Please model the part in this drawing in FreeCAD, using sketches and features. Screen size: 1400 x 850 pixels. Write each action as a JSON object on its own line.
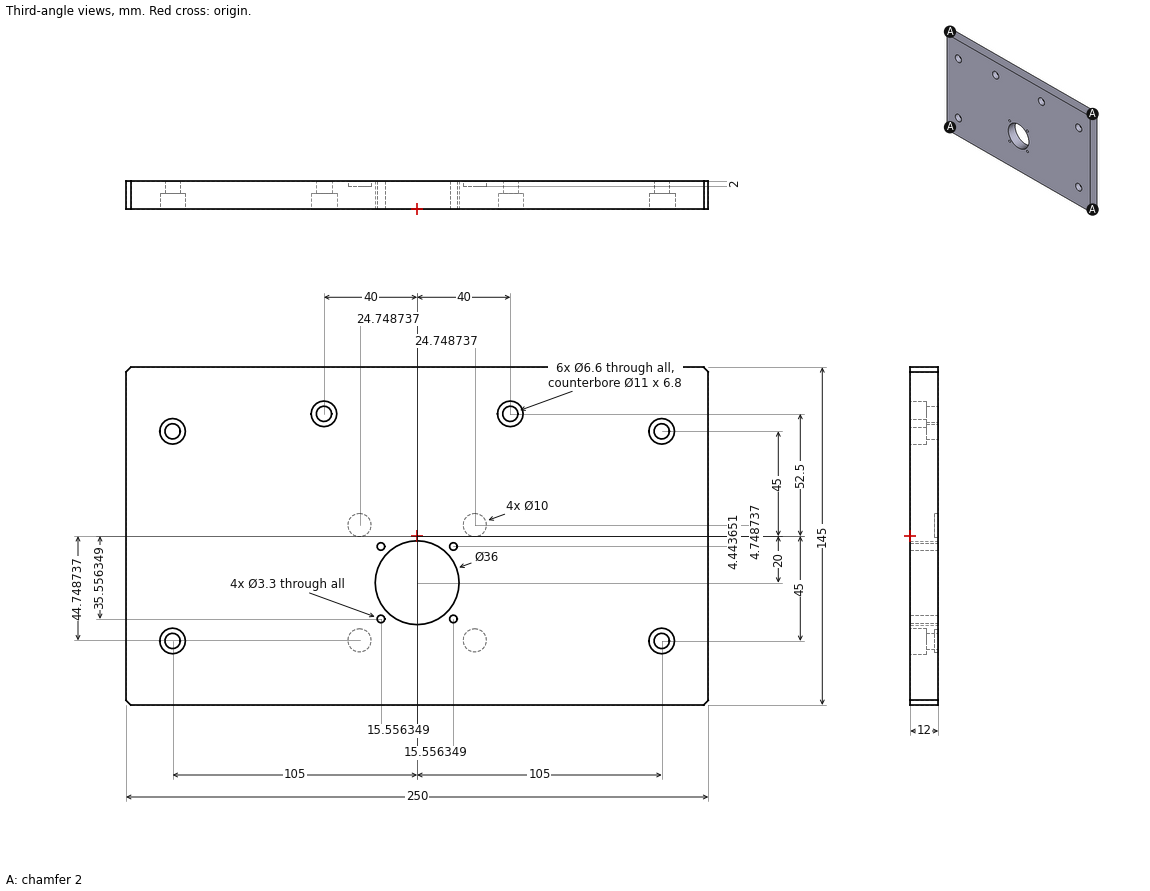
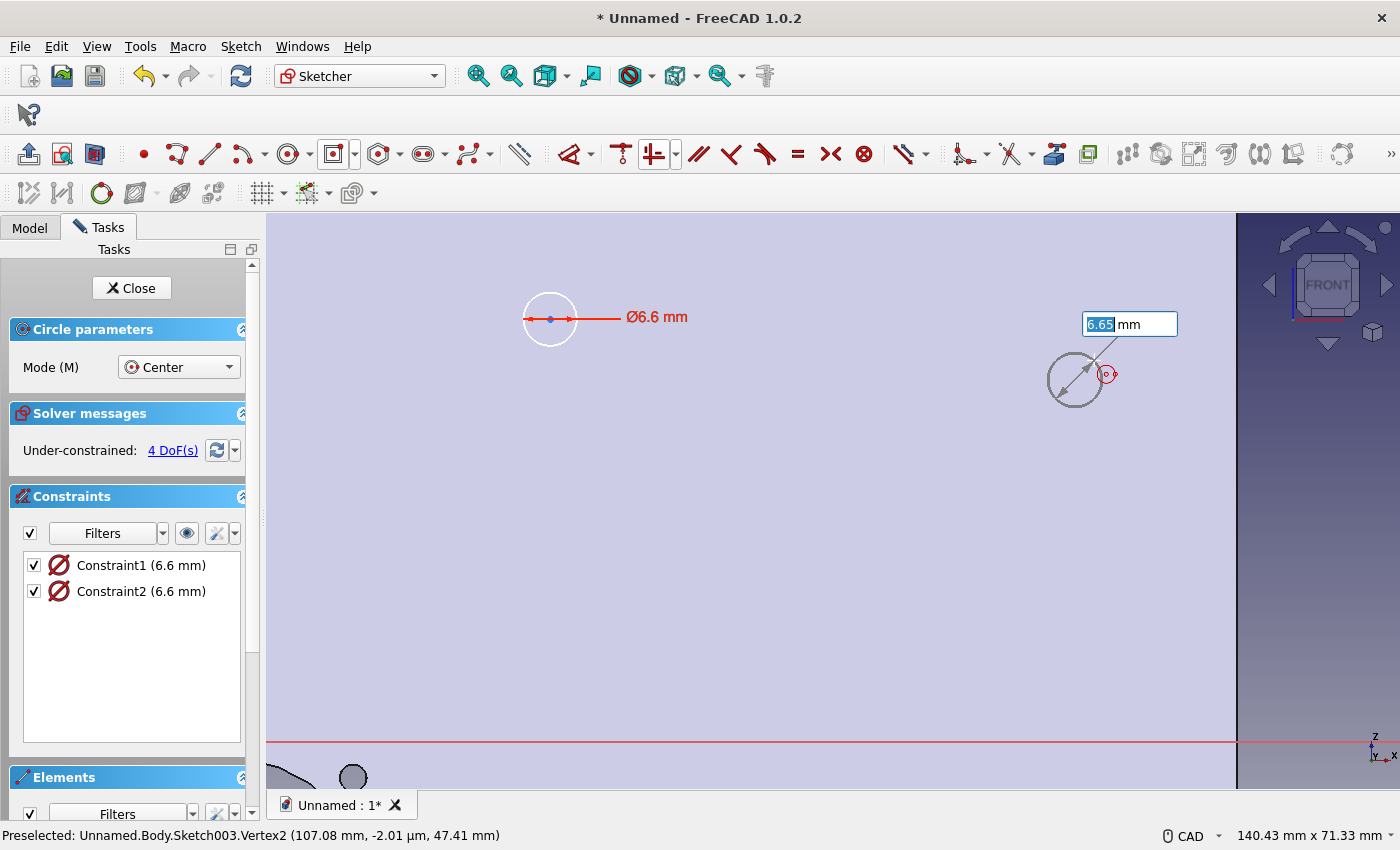
{"action": "type", "text": "6.6"}
{"action": "key", "text": "Return"}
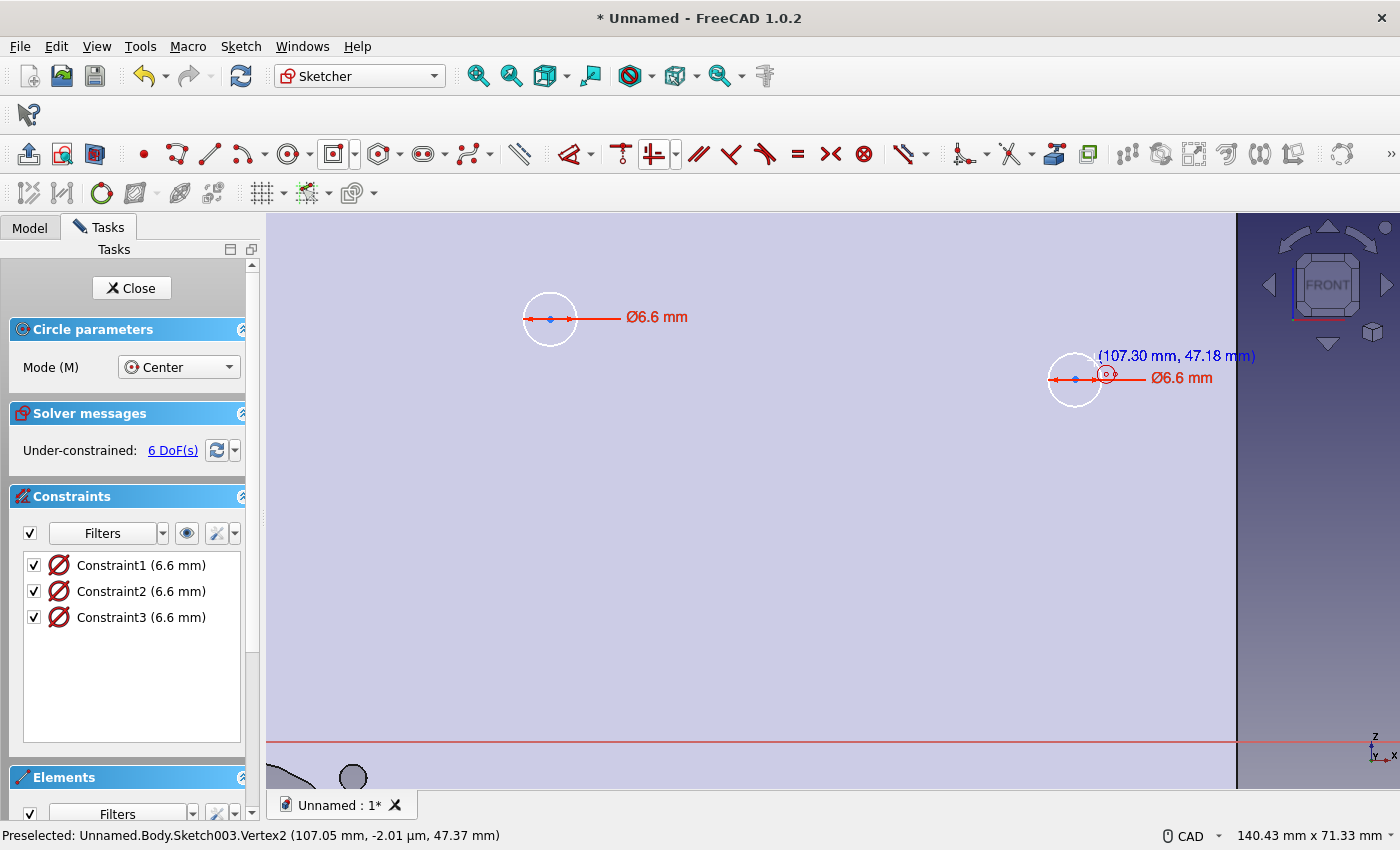
{"action": "scroll", "coordinate": [1077, 378], "scroll_direction": "down", "scroll_amount": 5}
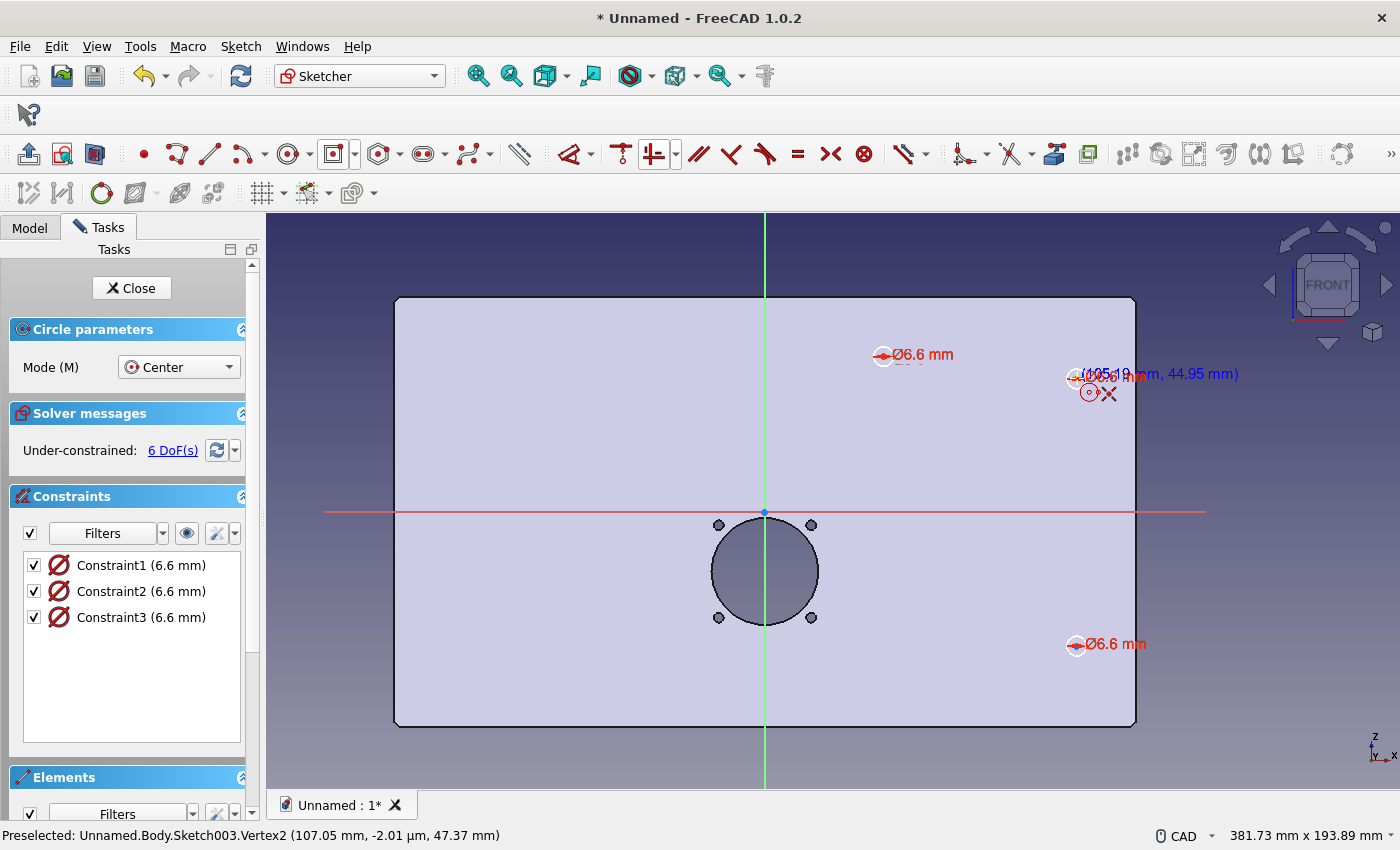
{"action": "scroll", "coordinate": [453, 646], "scroll_direction": "up", "scroll_amount": 5}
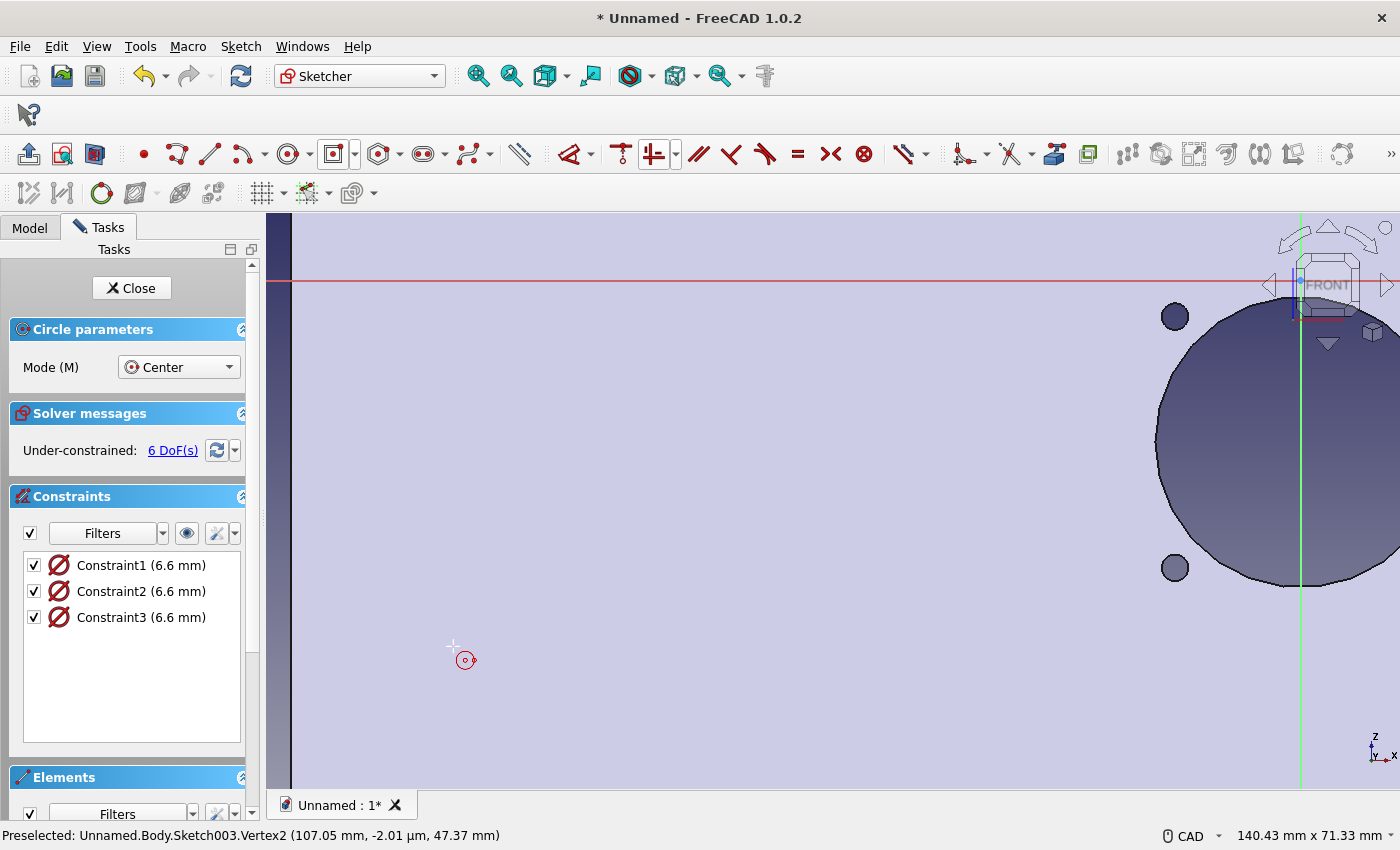
{"action": "left_click", "coordinate": [453, 644]}
{"action": "mouse_move", "coordinate": [472, 625]}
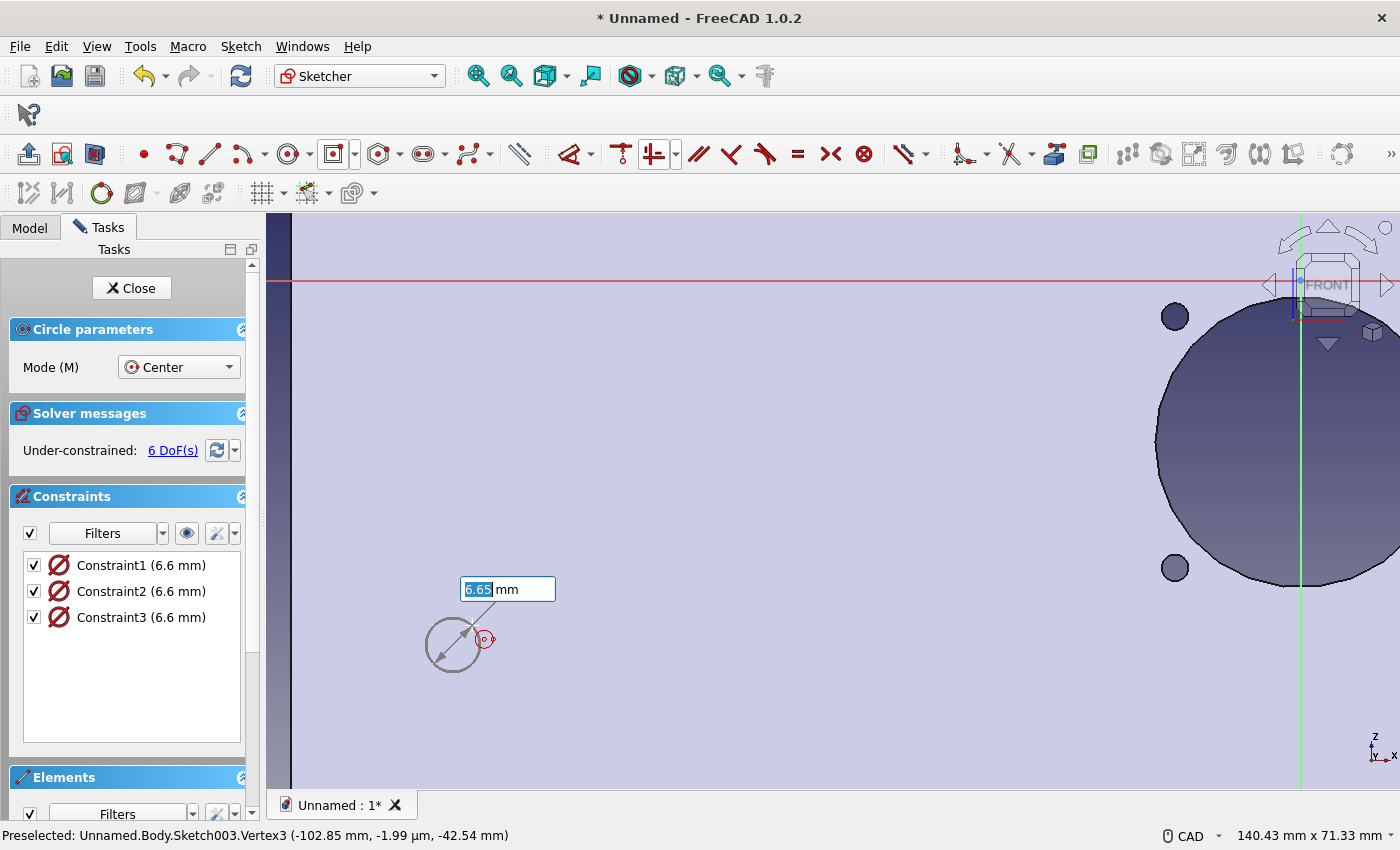
{"action": "type", "text": "6.6"}
{"action": "key", "text": "Return"}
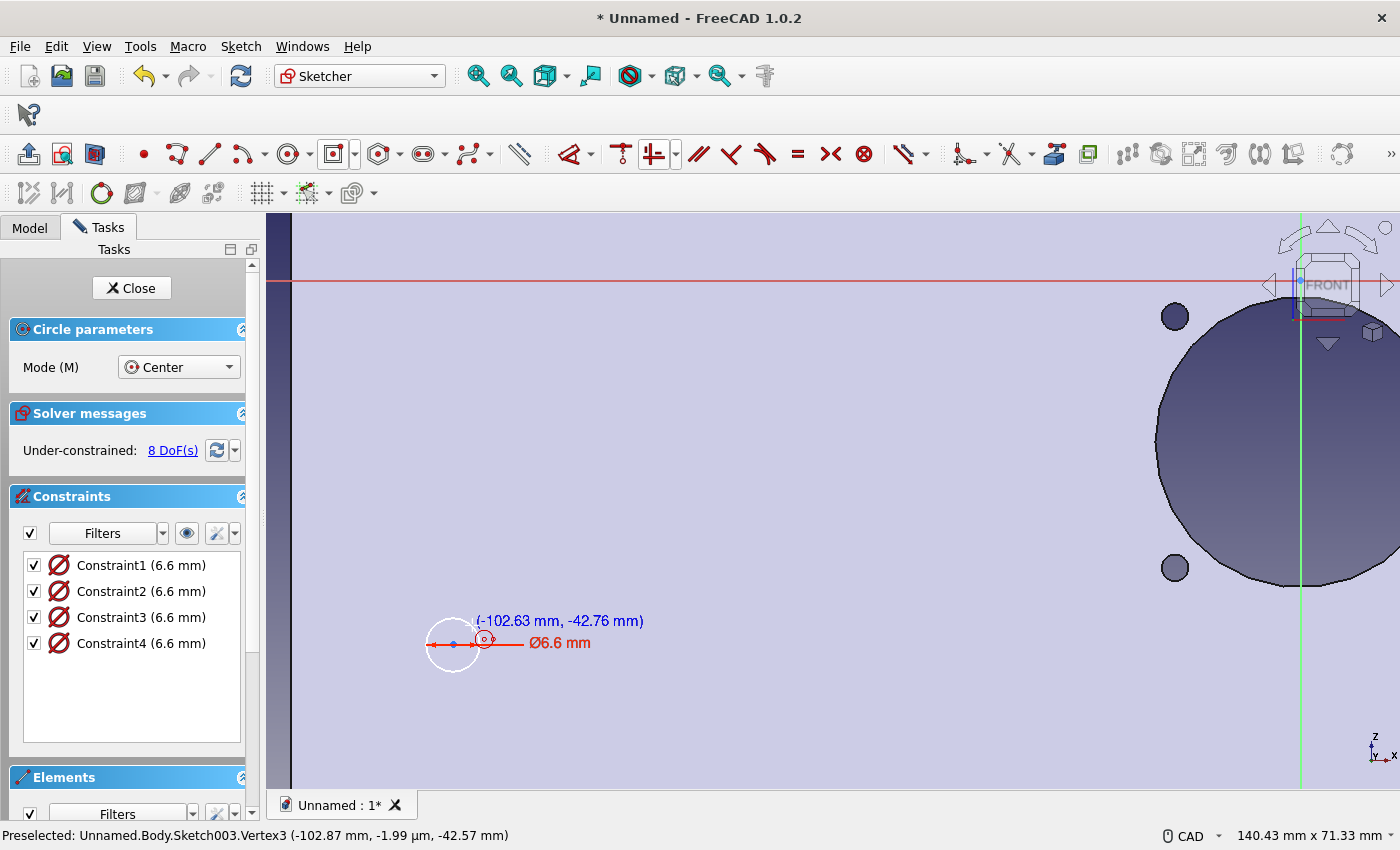
{"action": "scroll", "coordinate": [452, 647], "scroll_direction": "down", "scroll_amount": 5}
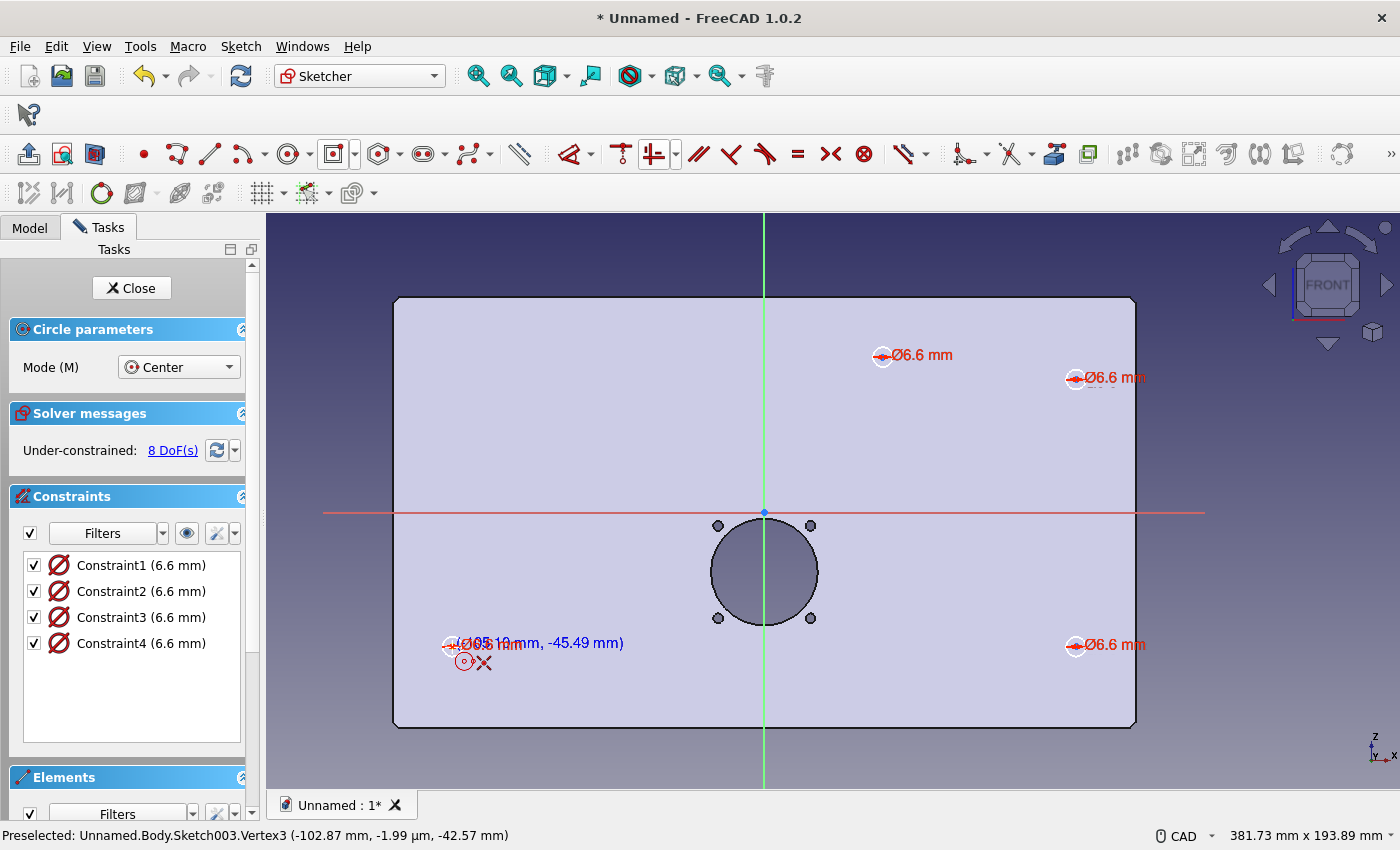
{"action": "scroll", "coordinate": [452, 379], "scroll_direction": "up", "scroll_amount": 5}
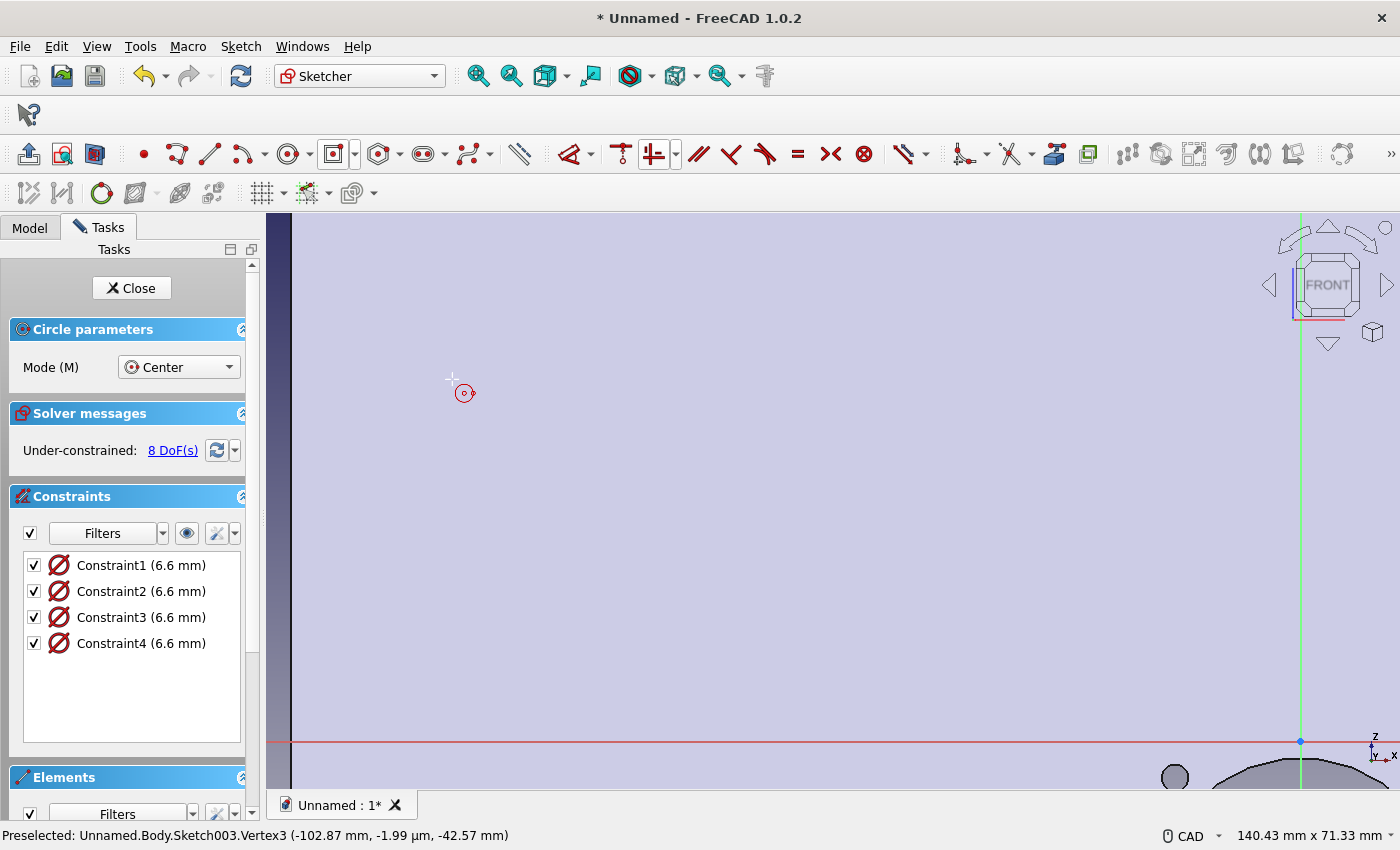
{"action": "left_click", "coordinate": [453, 379]}
{"action": "mouse_move", "coordinate": [472, 360]}